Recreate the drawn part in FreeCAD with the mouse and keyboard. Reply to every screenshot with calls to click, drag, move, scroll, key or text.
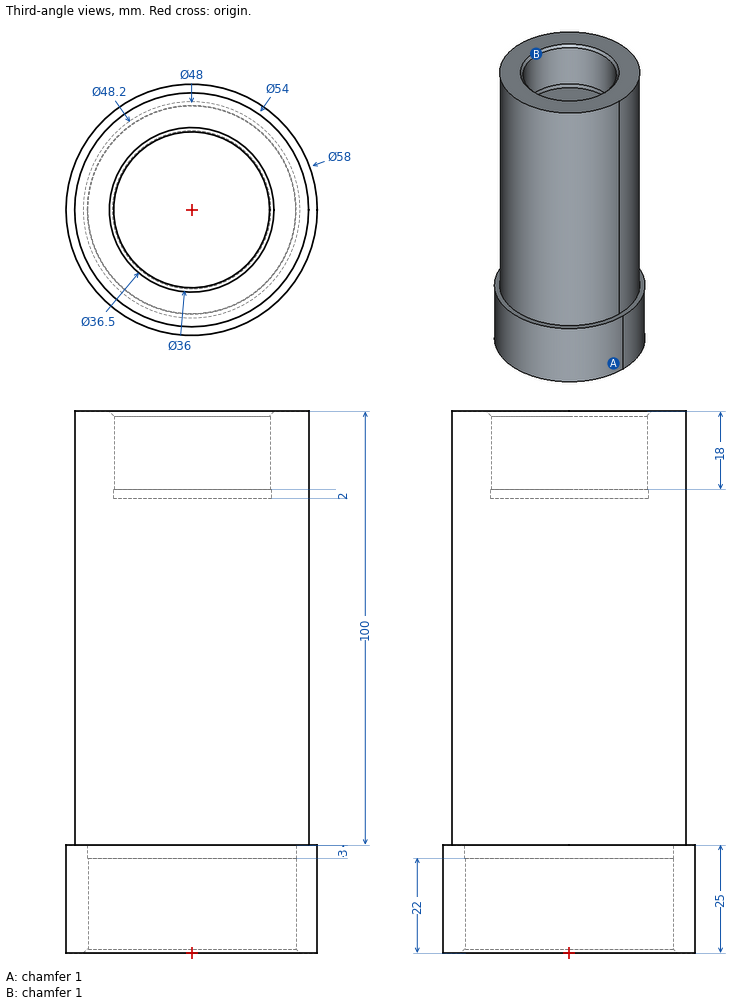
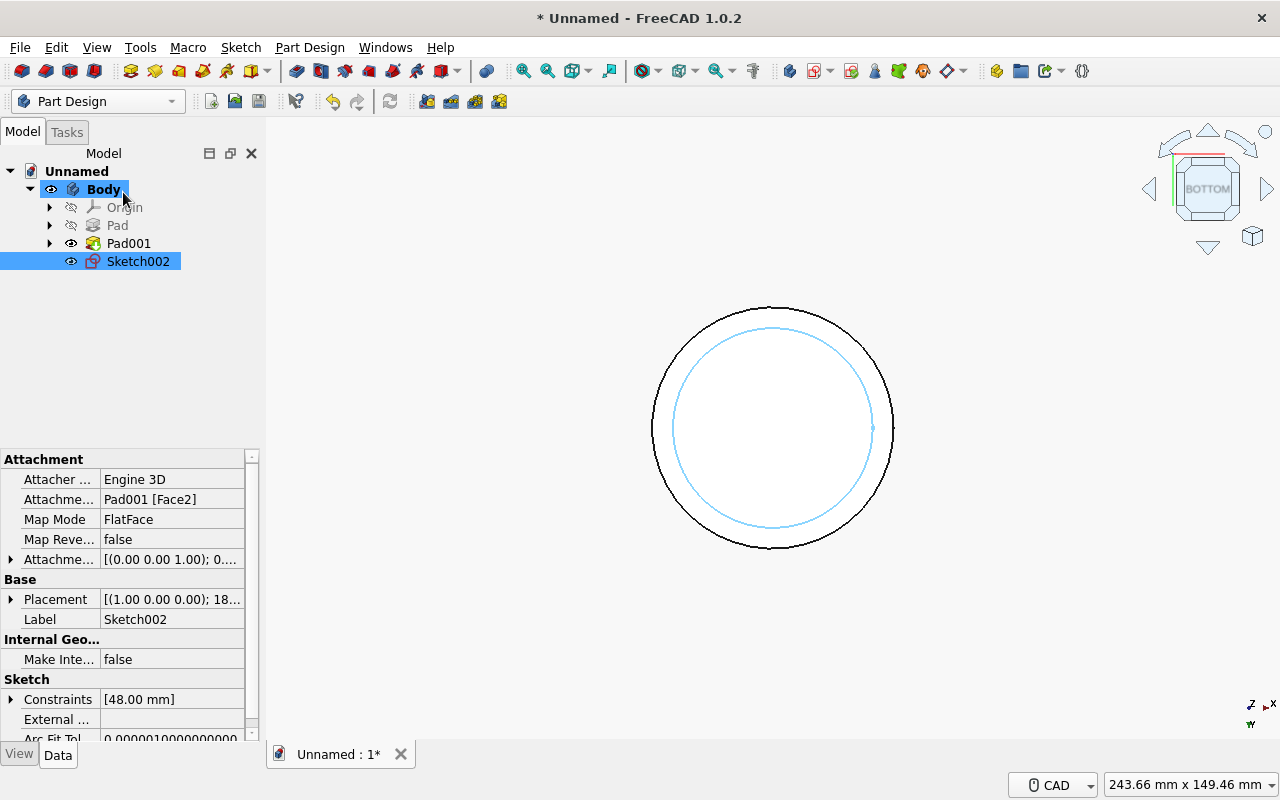
click(298, 72)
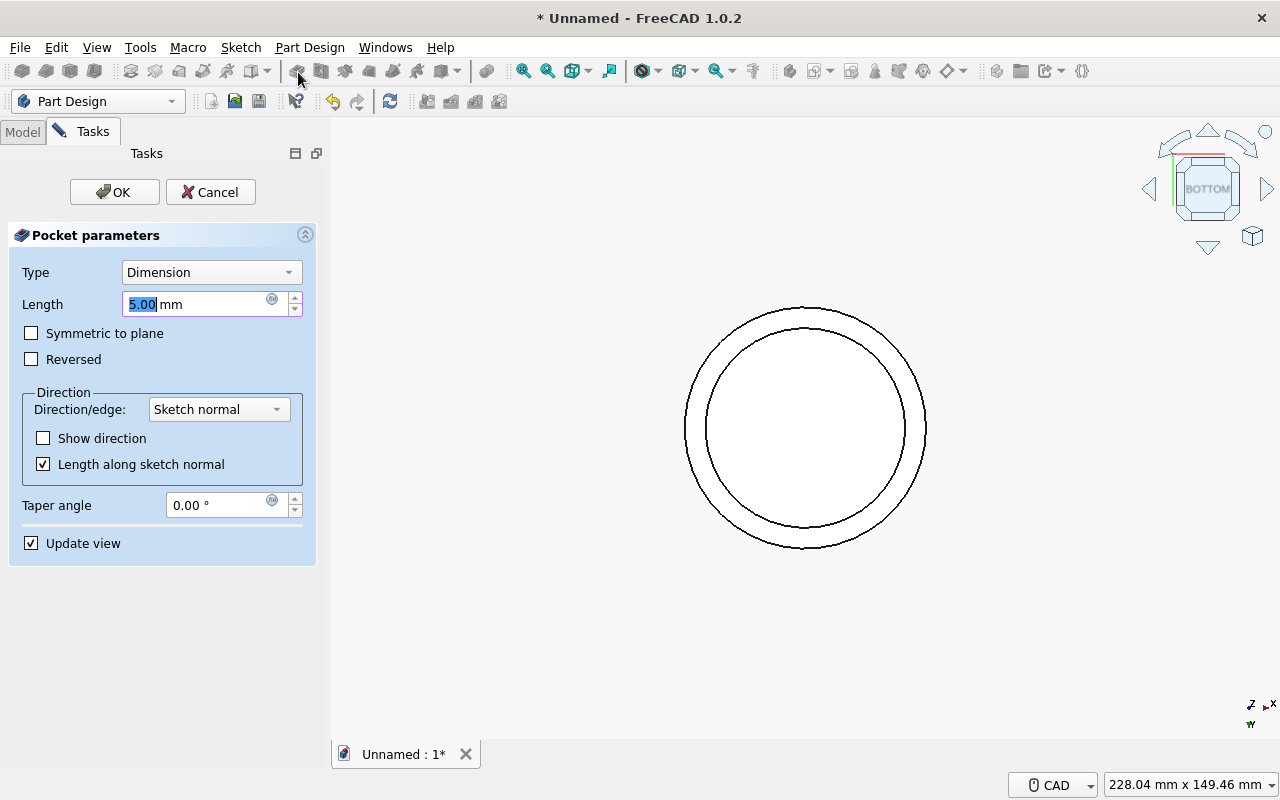
text(22)
key(Tab)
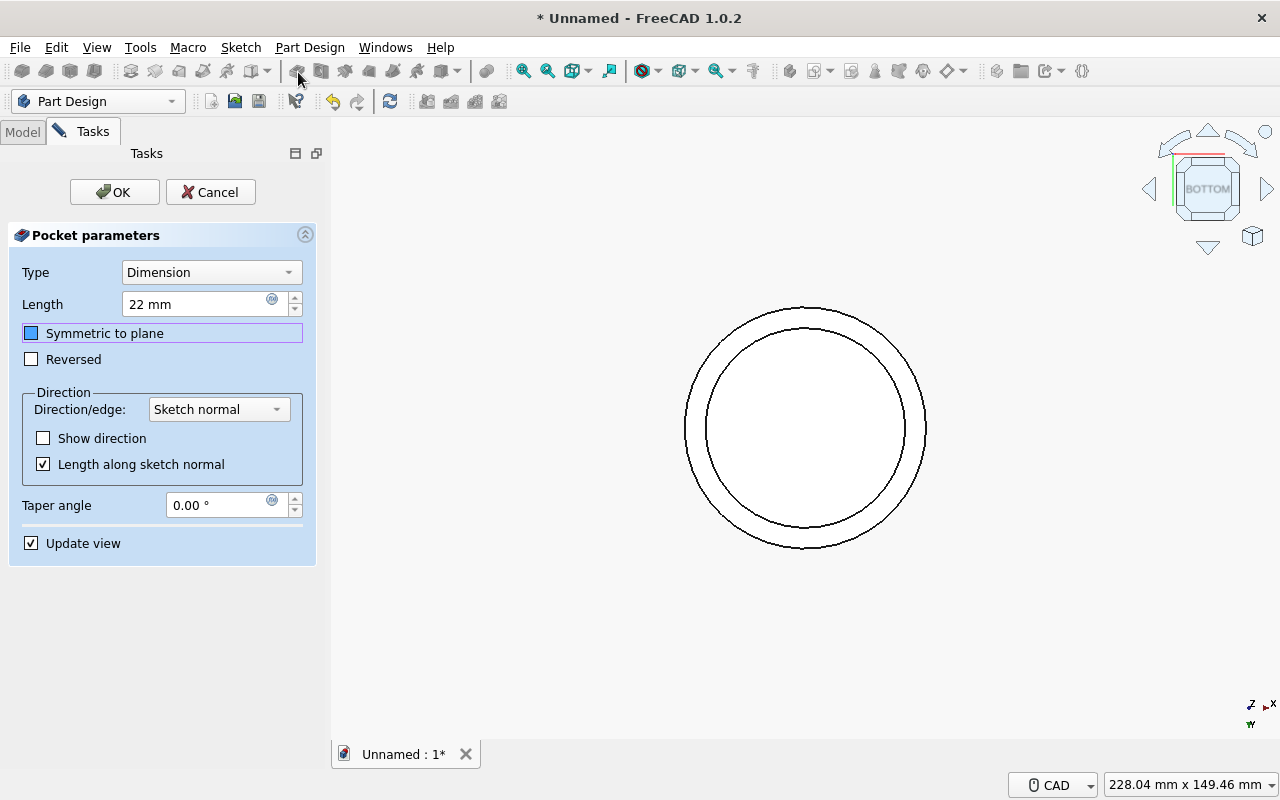
click(115, 192)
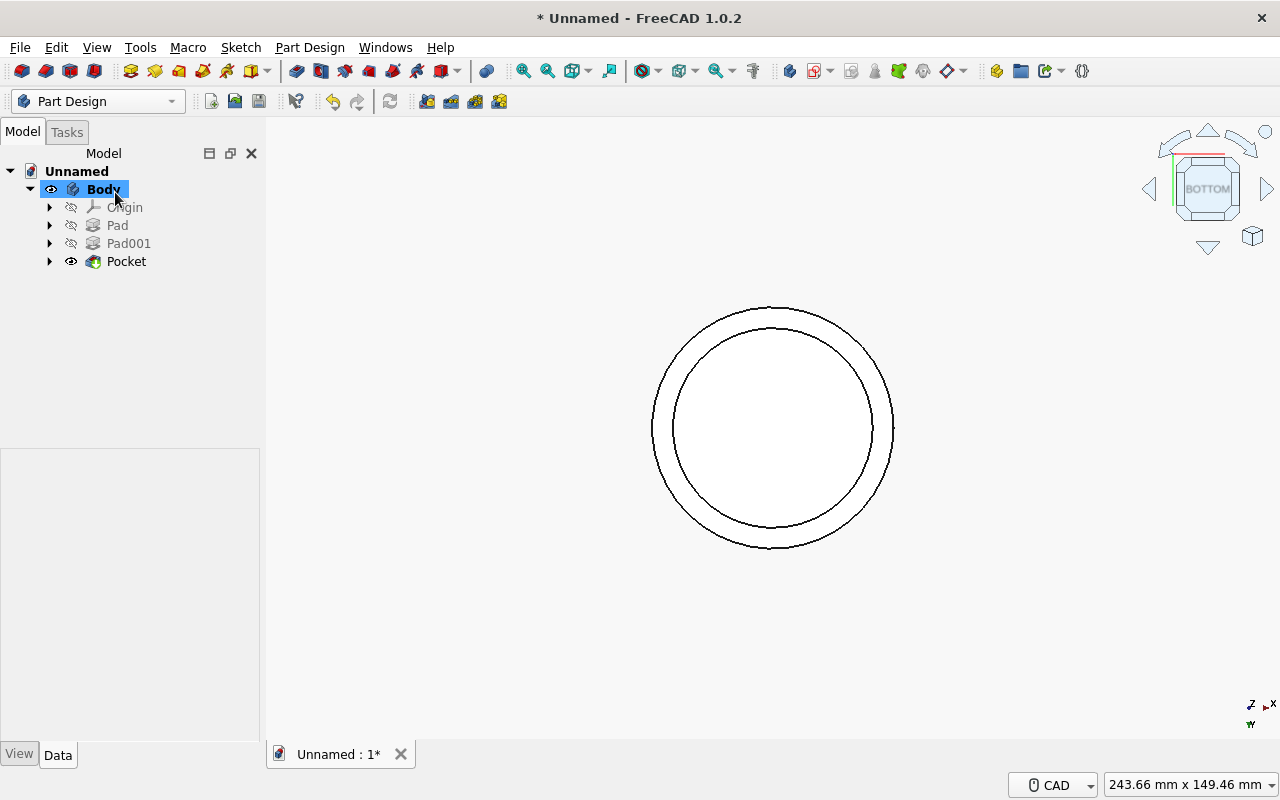
key(v)
key(f)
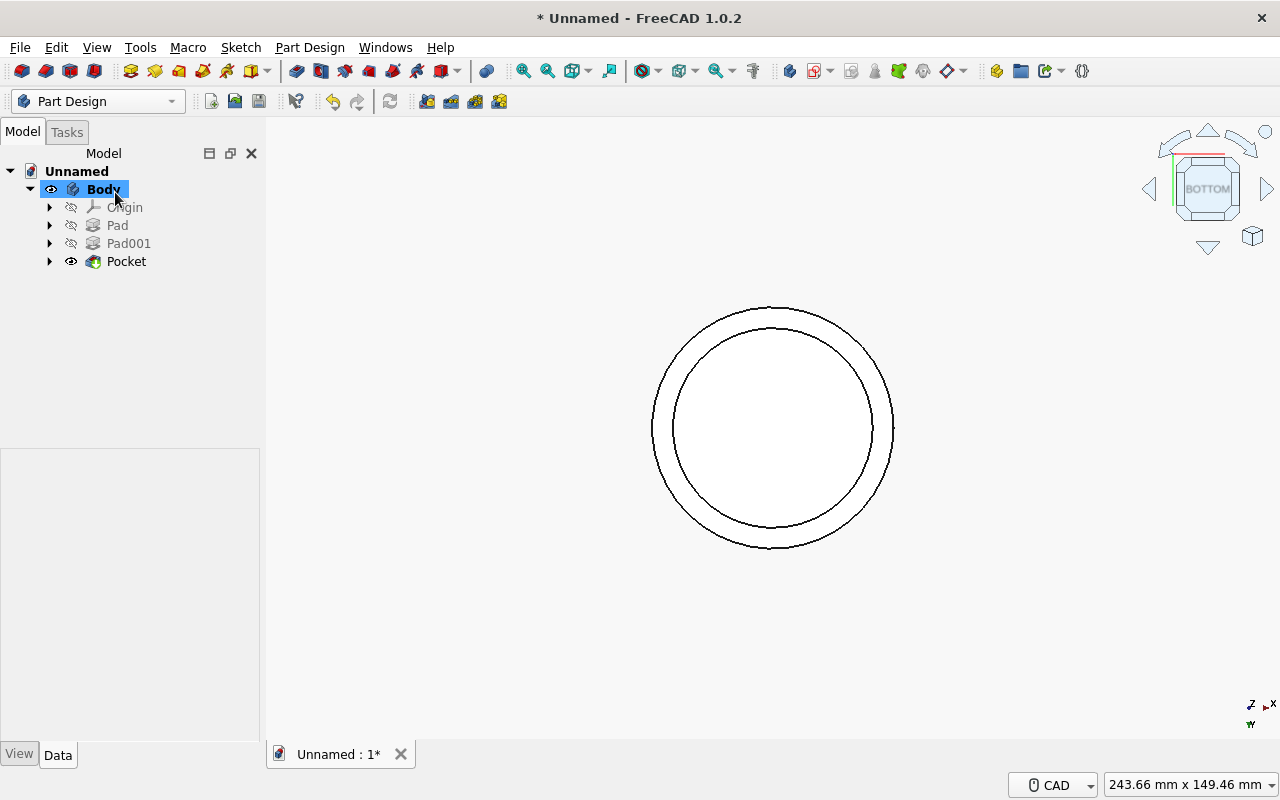
click(773, 427)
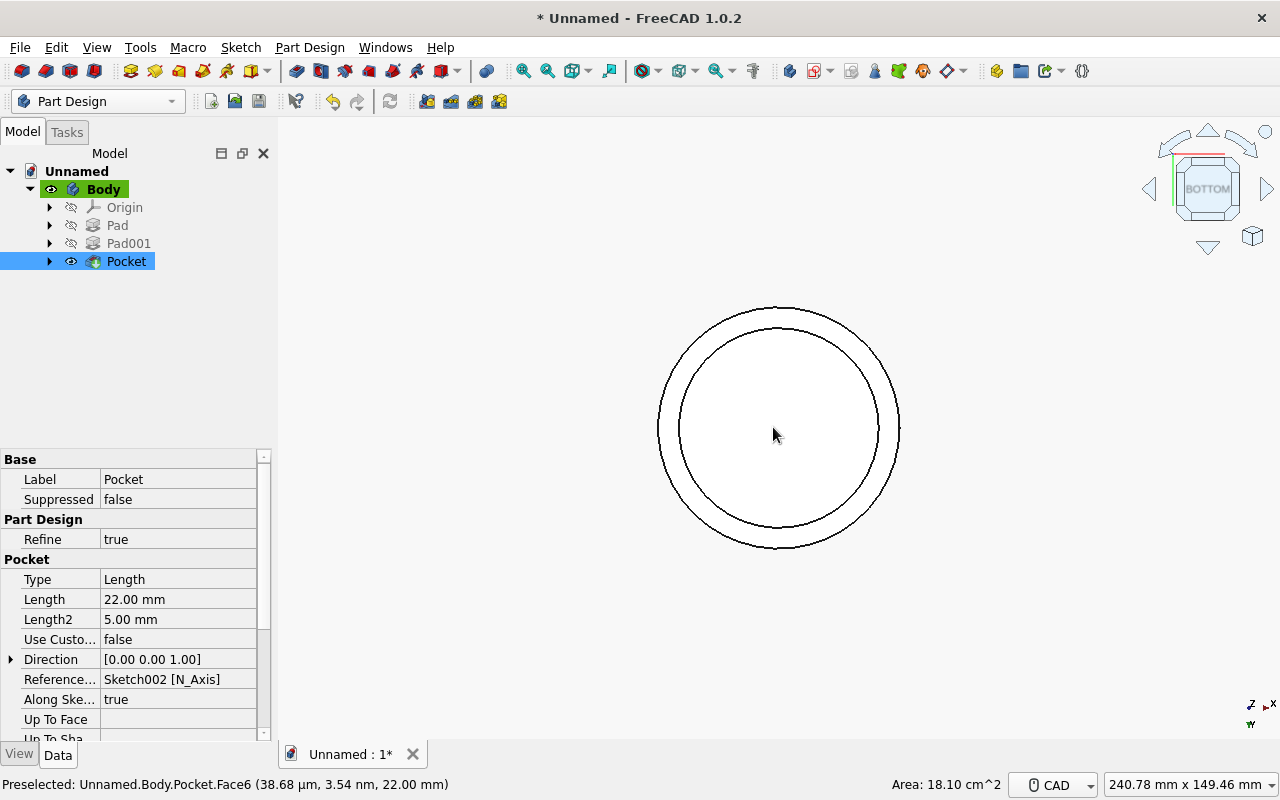
click(814, 72)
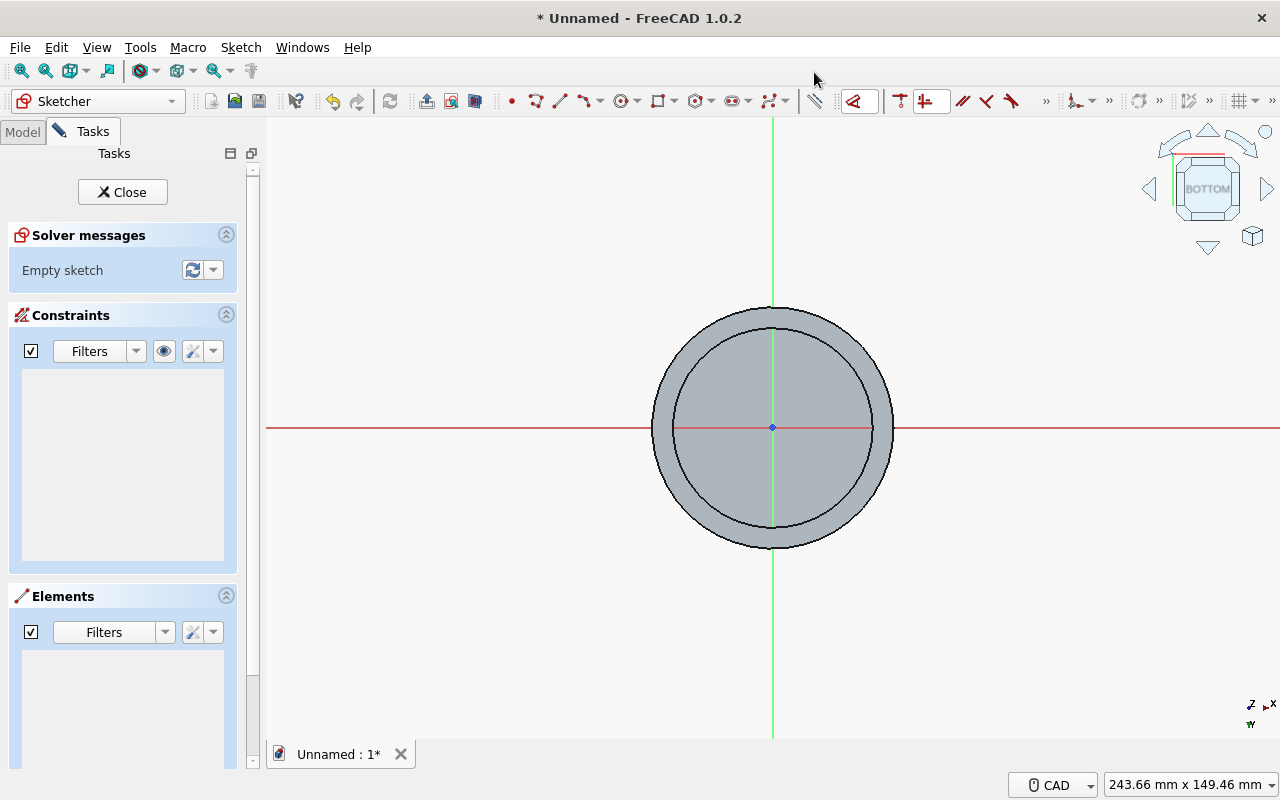
scroll(856, 428, up, 3)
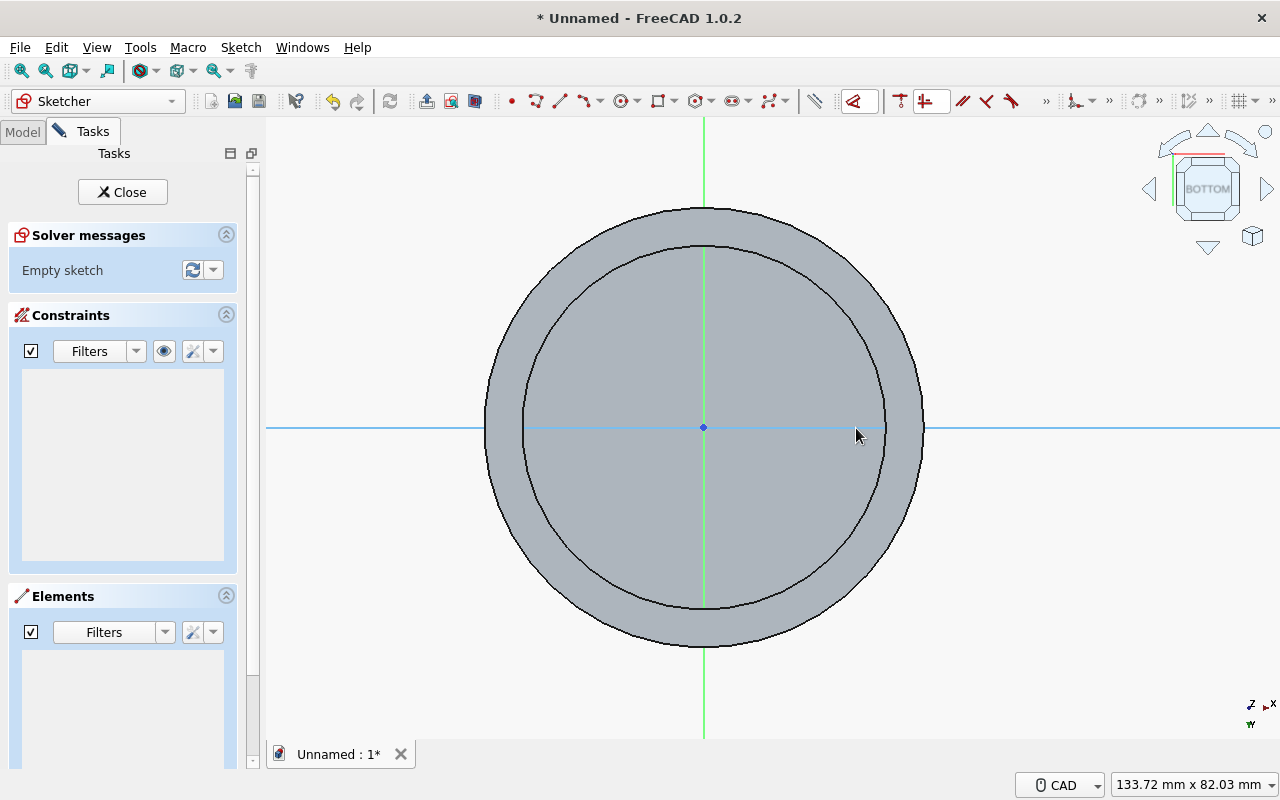
click(622, 102)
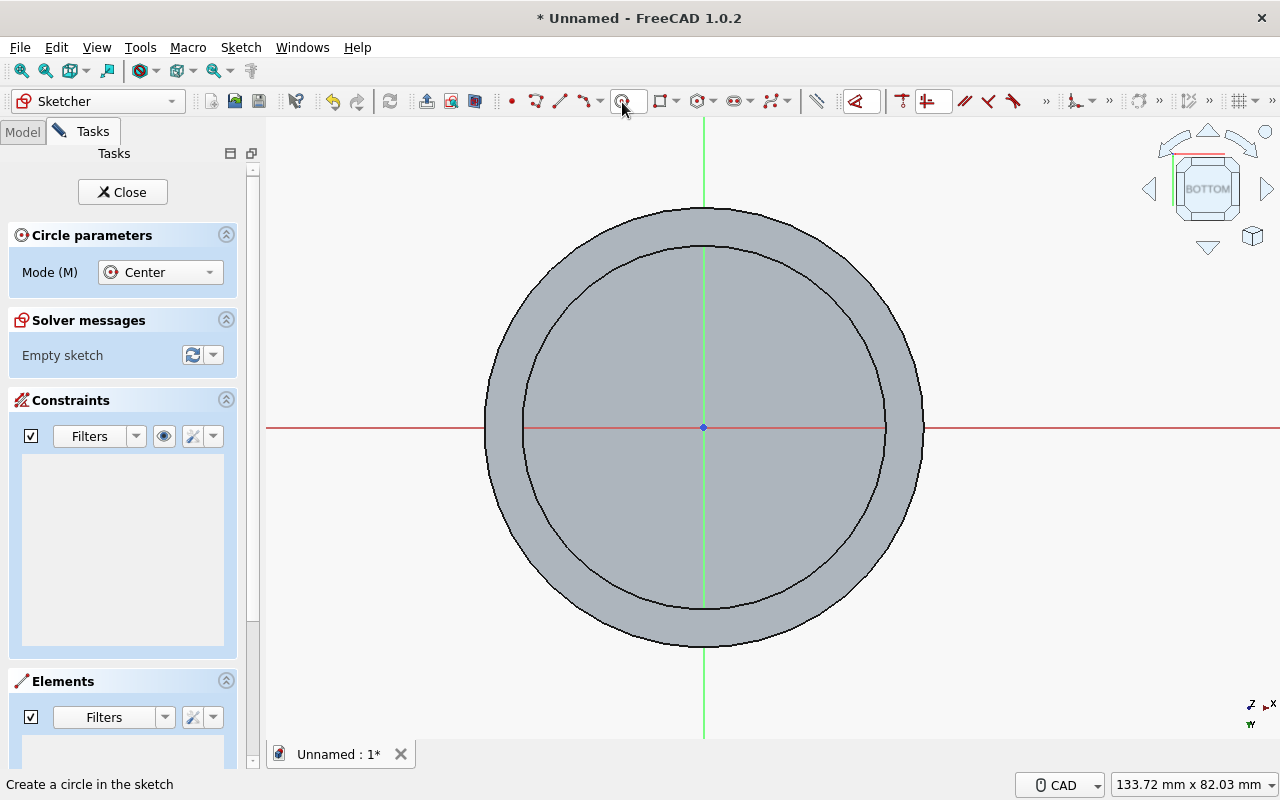
click(704, 428)
move(833, 298)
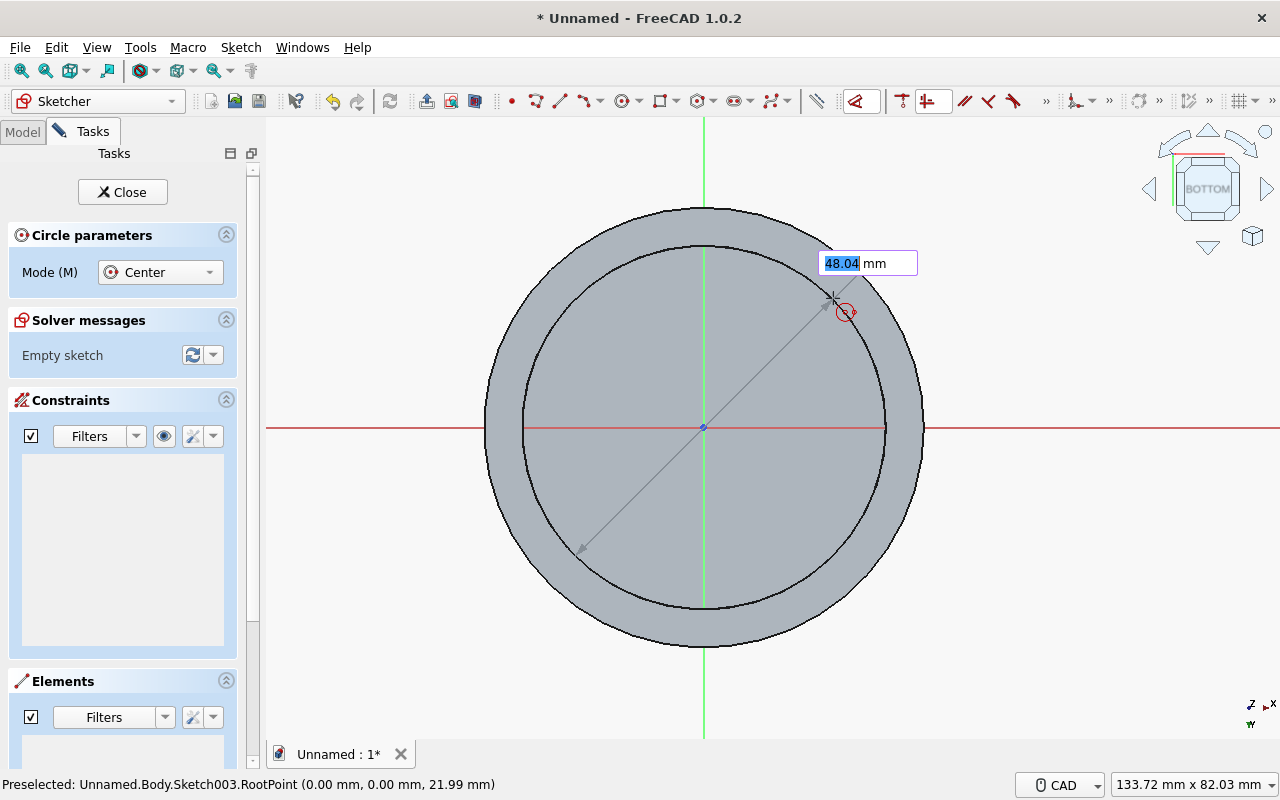
text(48.2)
key(Return)
key(Escape)